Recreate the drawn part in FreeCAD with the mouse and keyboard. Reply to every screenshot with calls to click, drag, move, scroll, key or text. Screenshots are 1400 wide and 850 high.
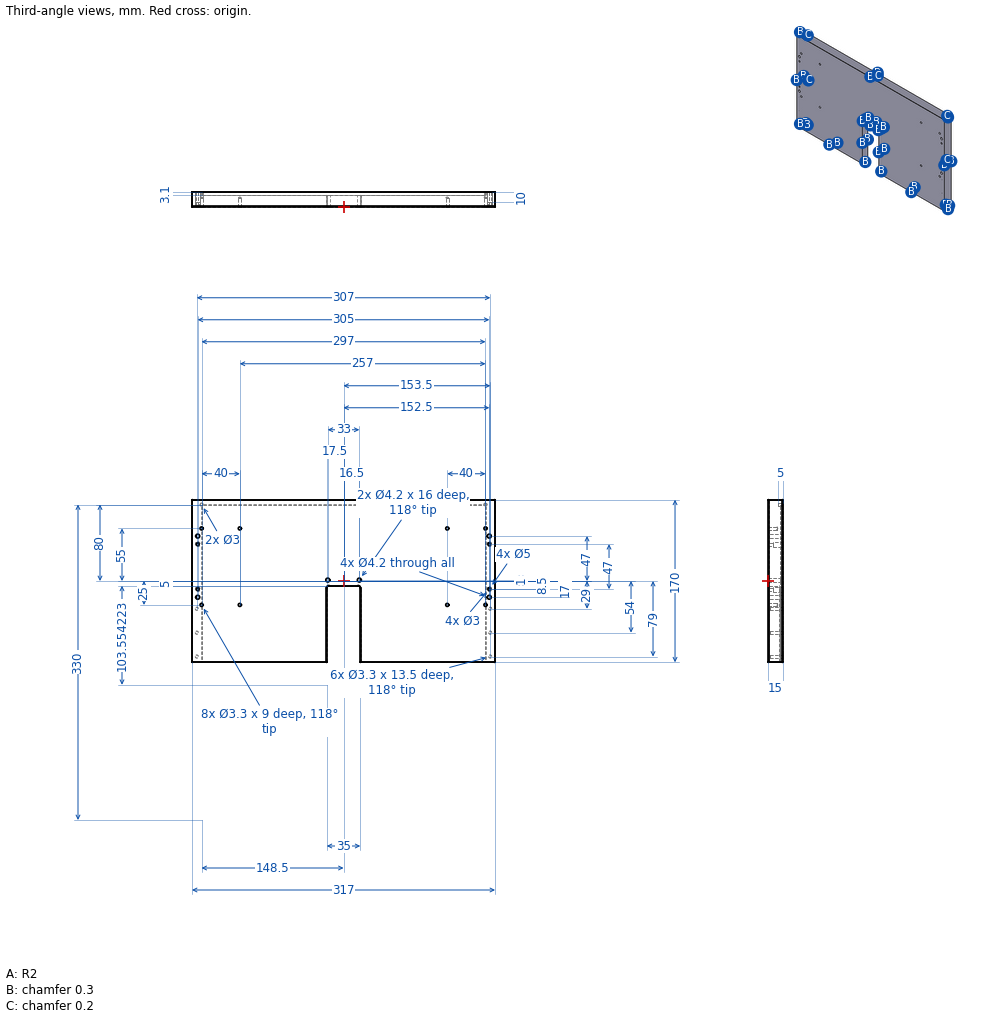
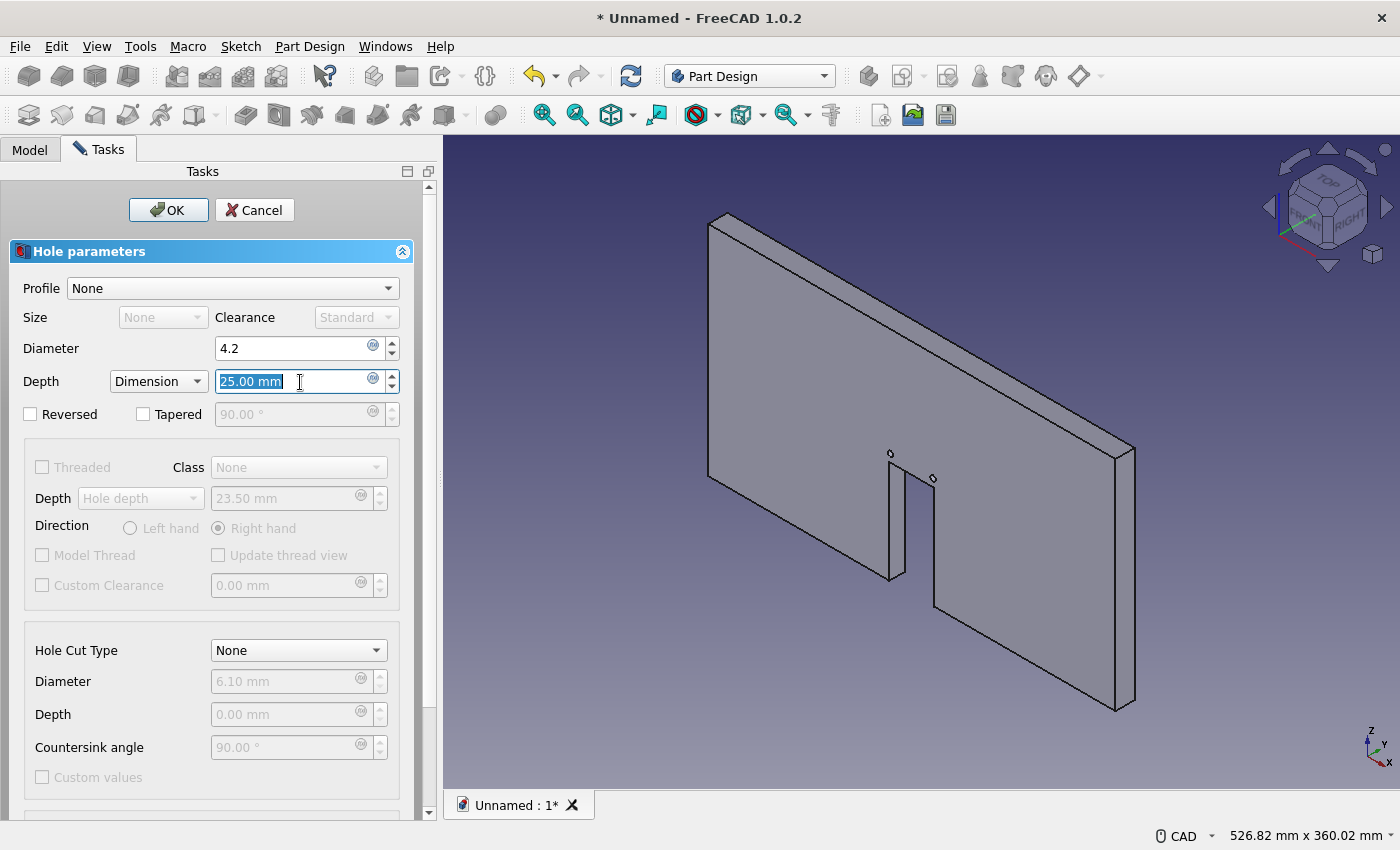
text(16)
key(Tab)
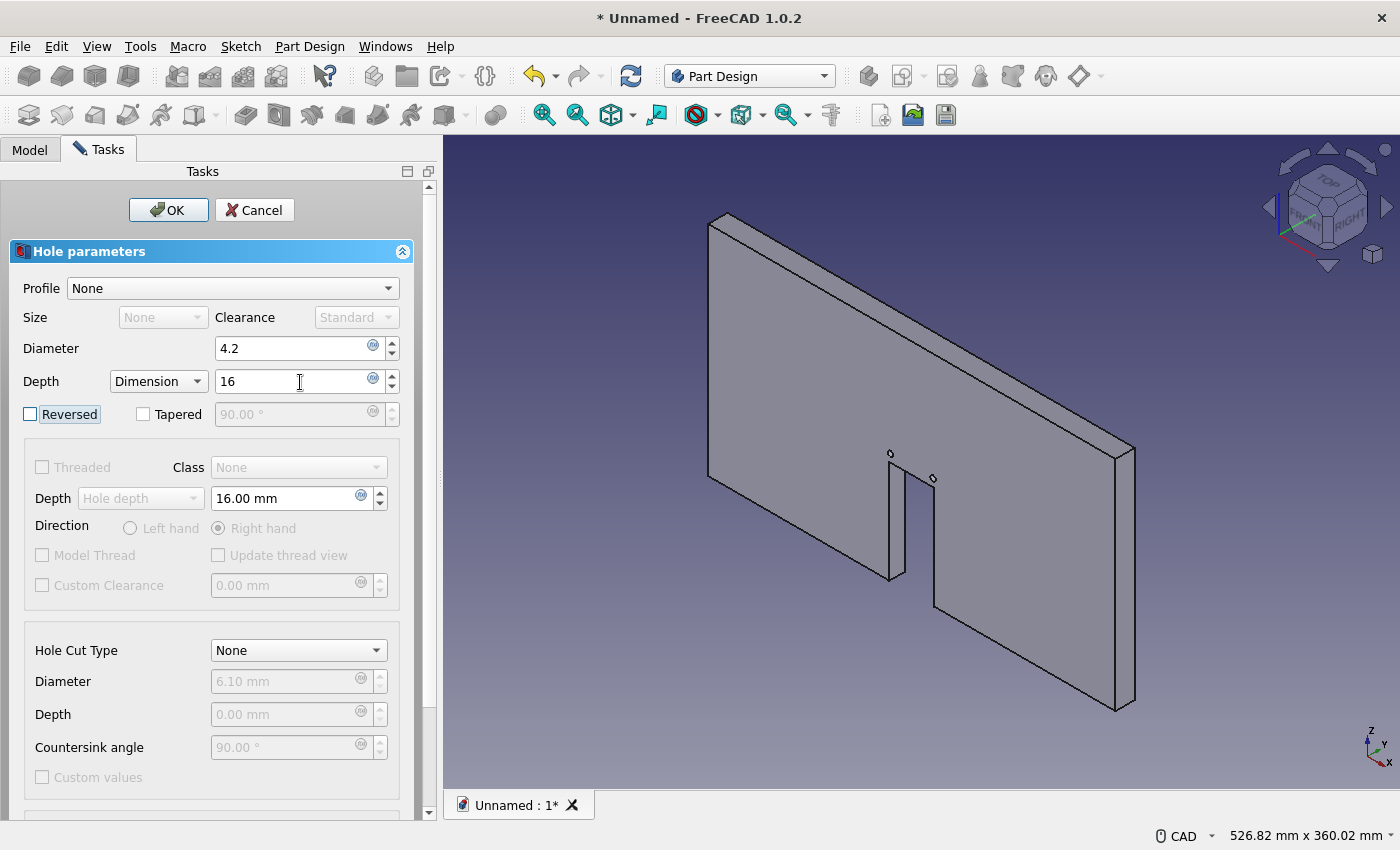
click(169, 210)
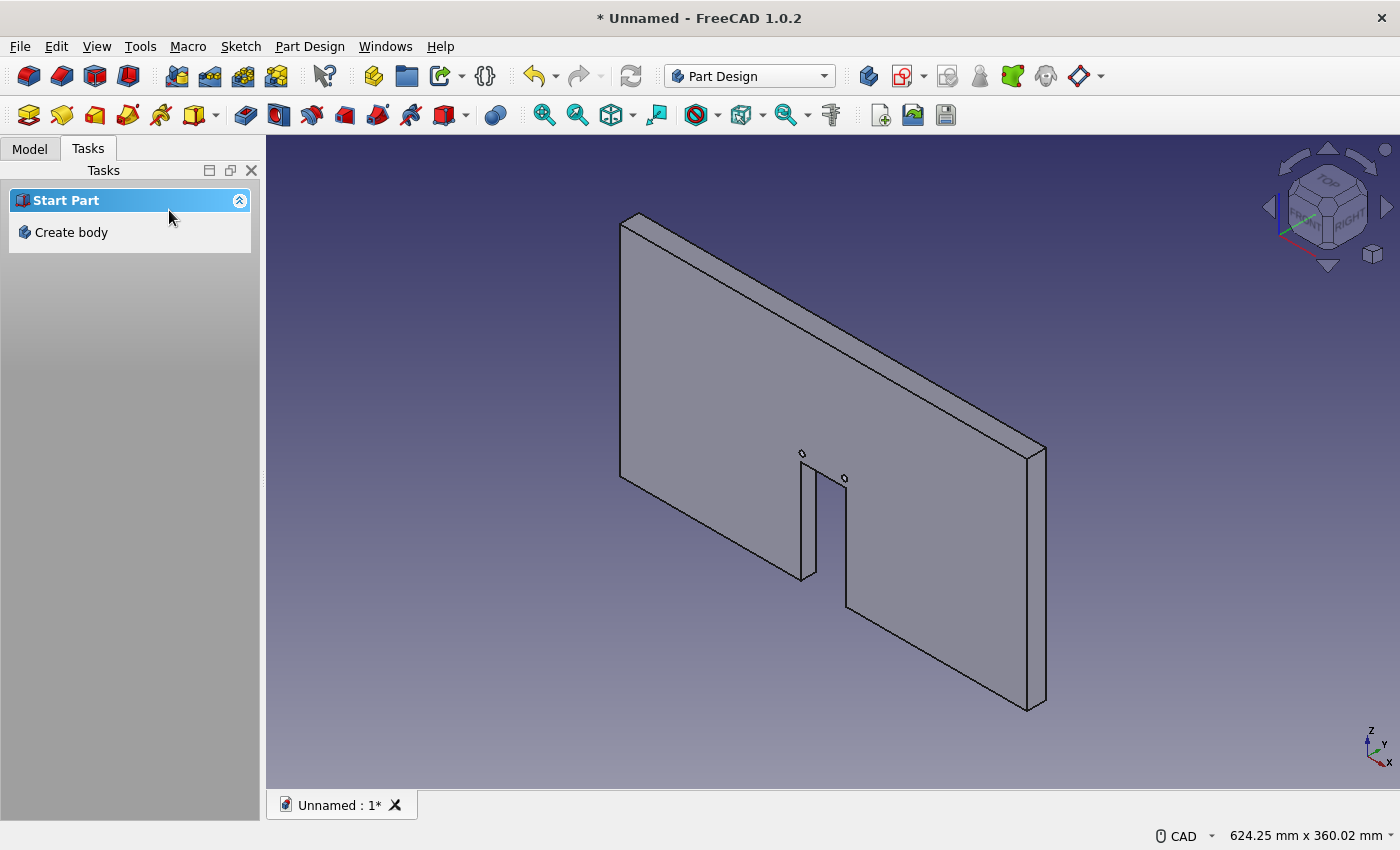
scroll(853, 483, up, 4)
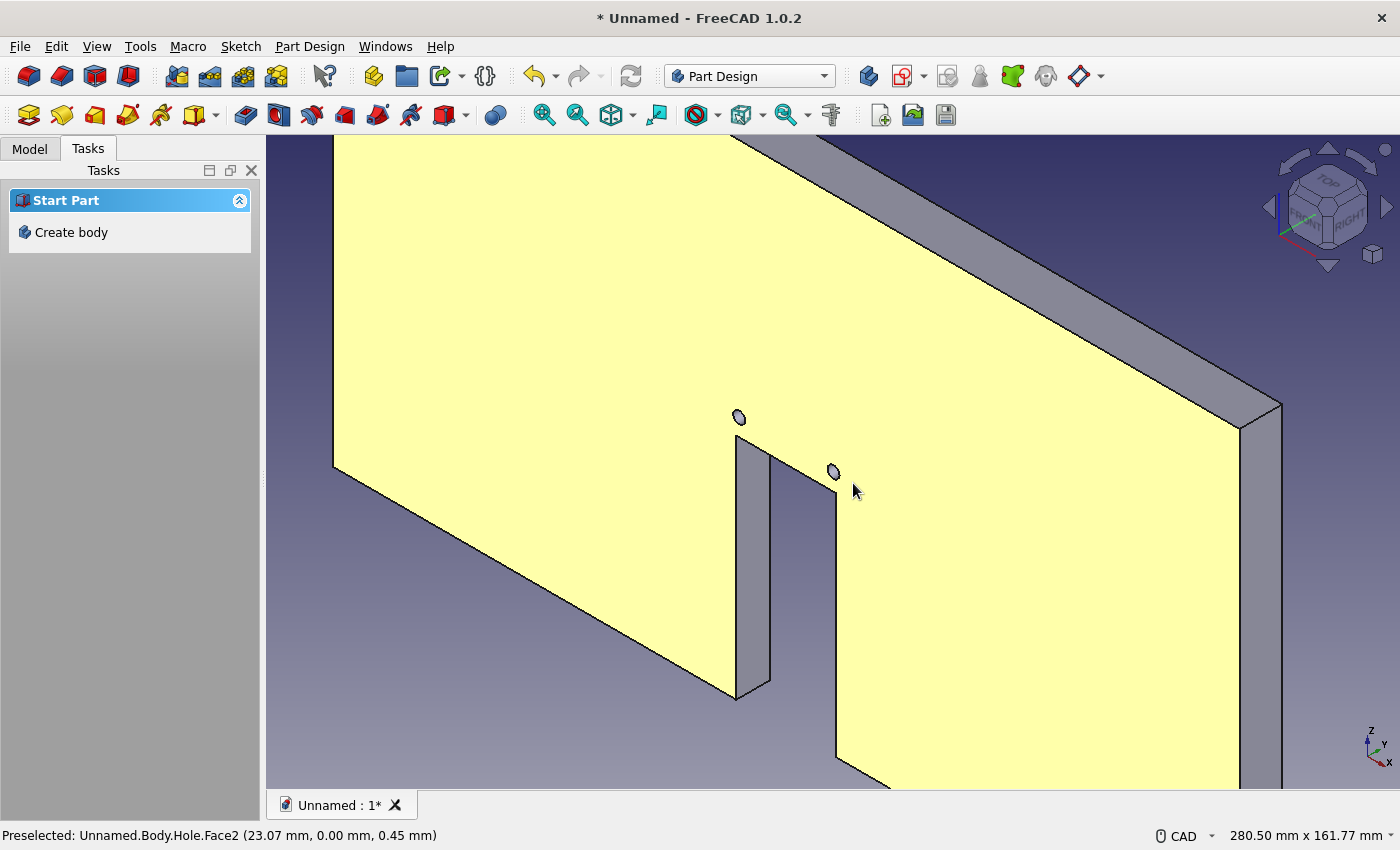
key(v)
key(f)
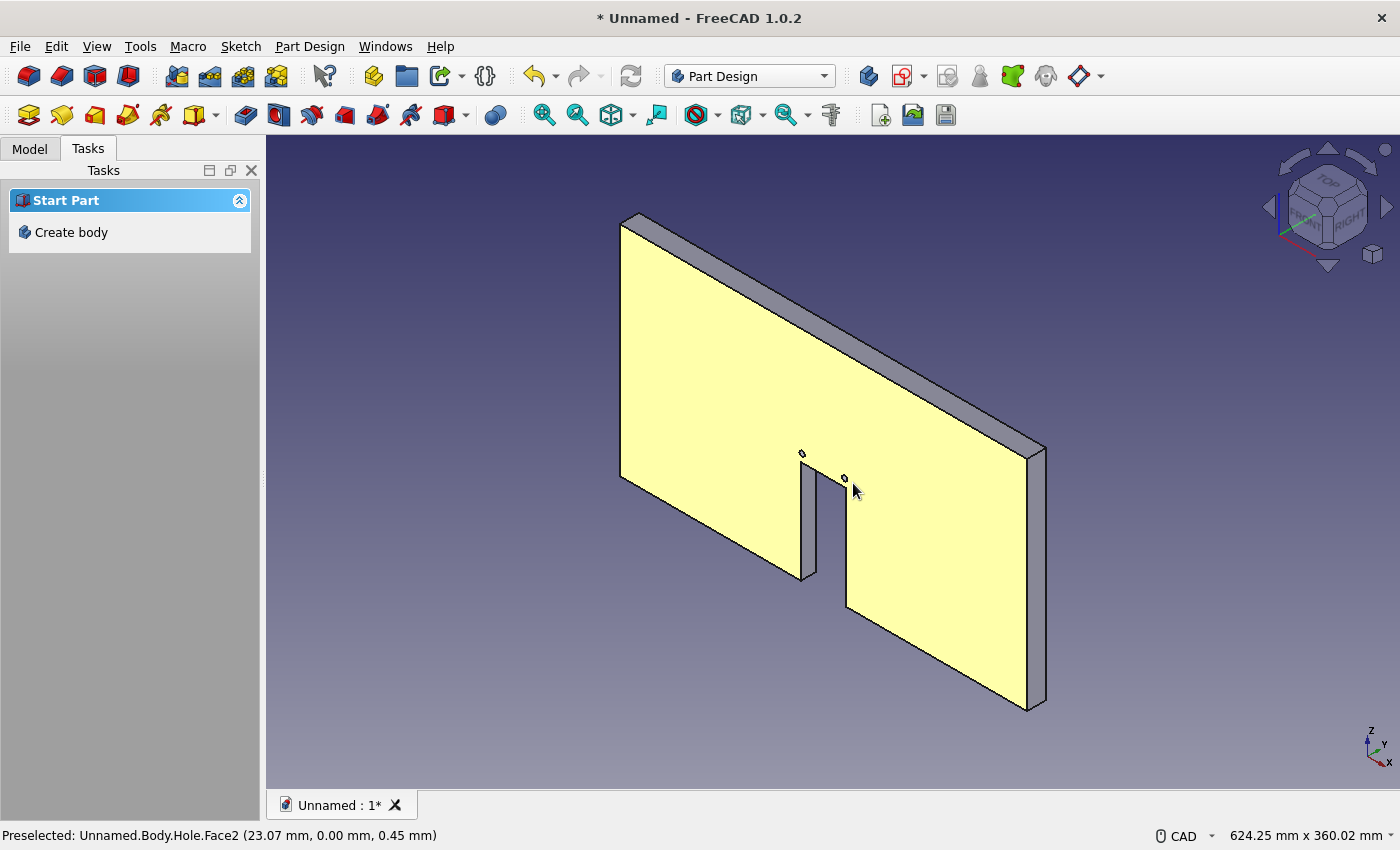
key(2)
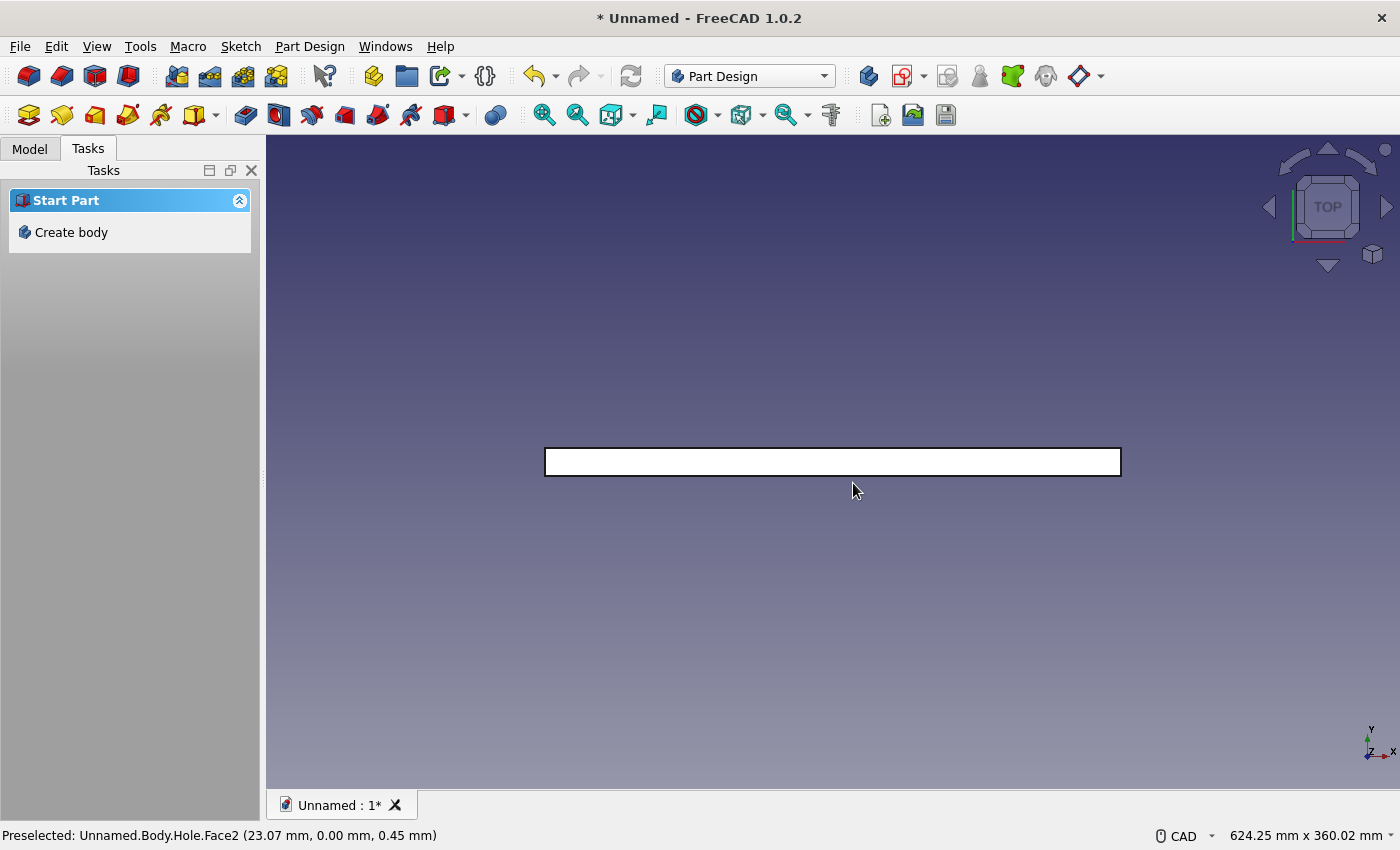
scroll(865, 464, up, 4)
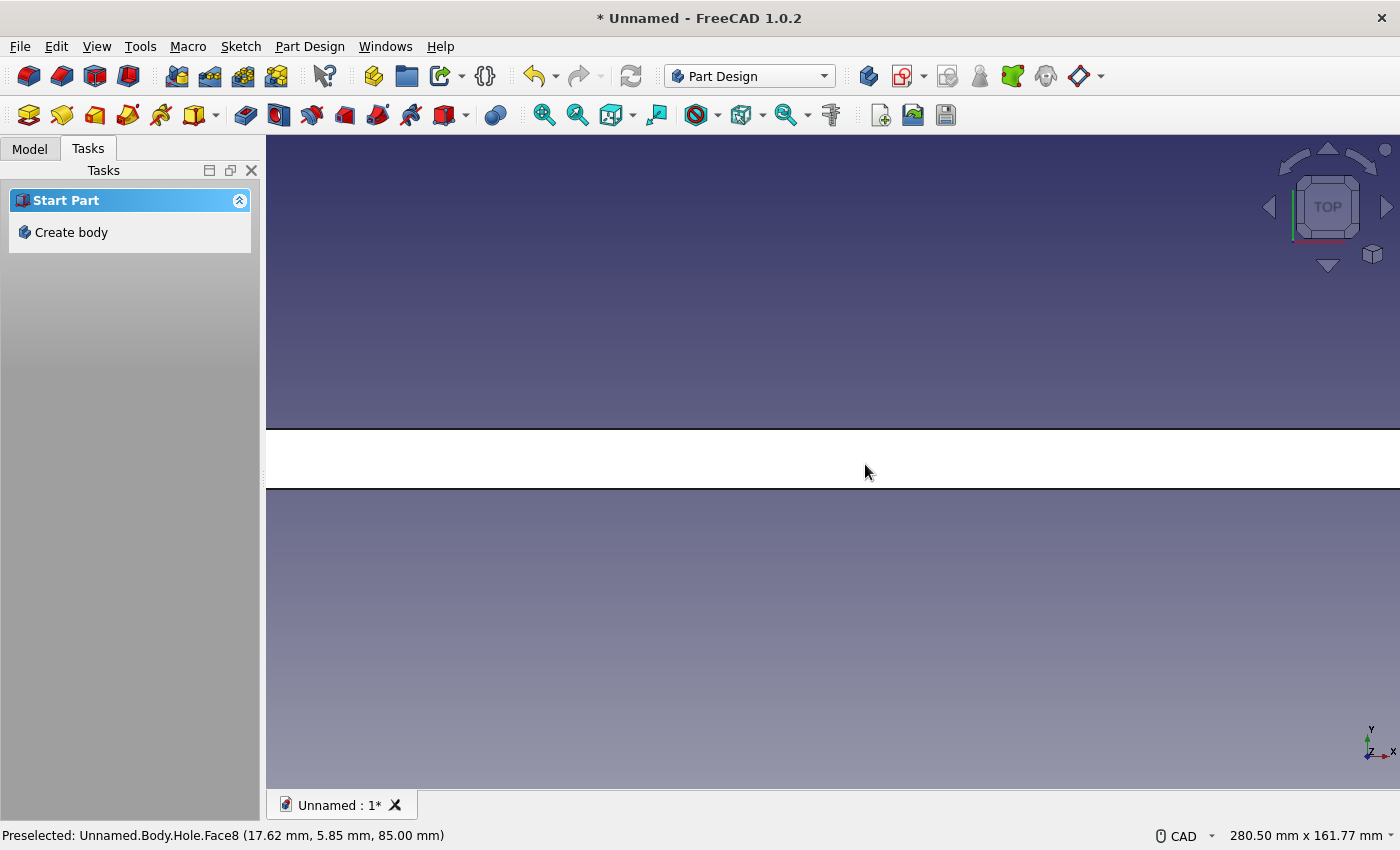
click(545, 116)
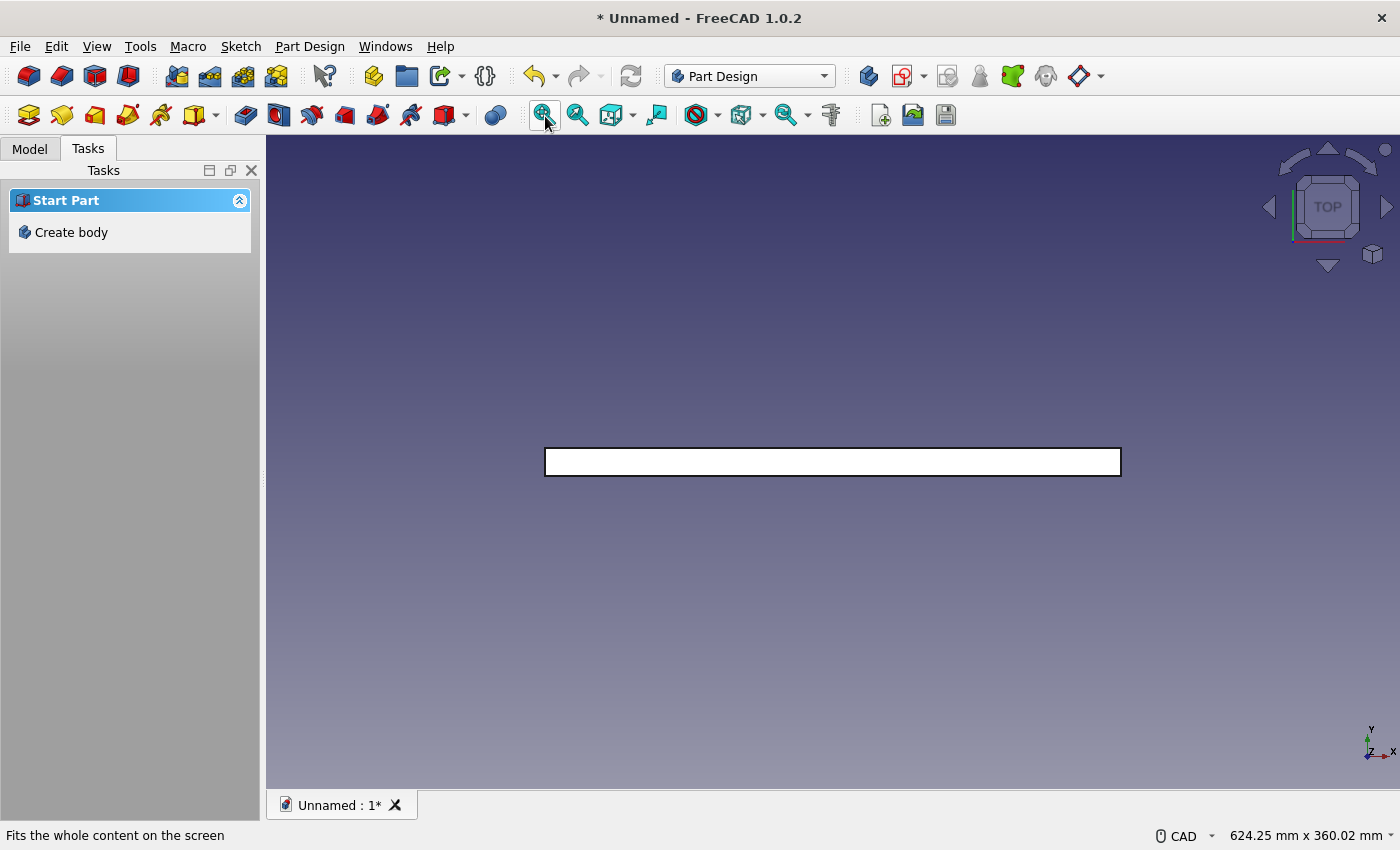
key(0)